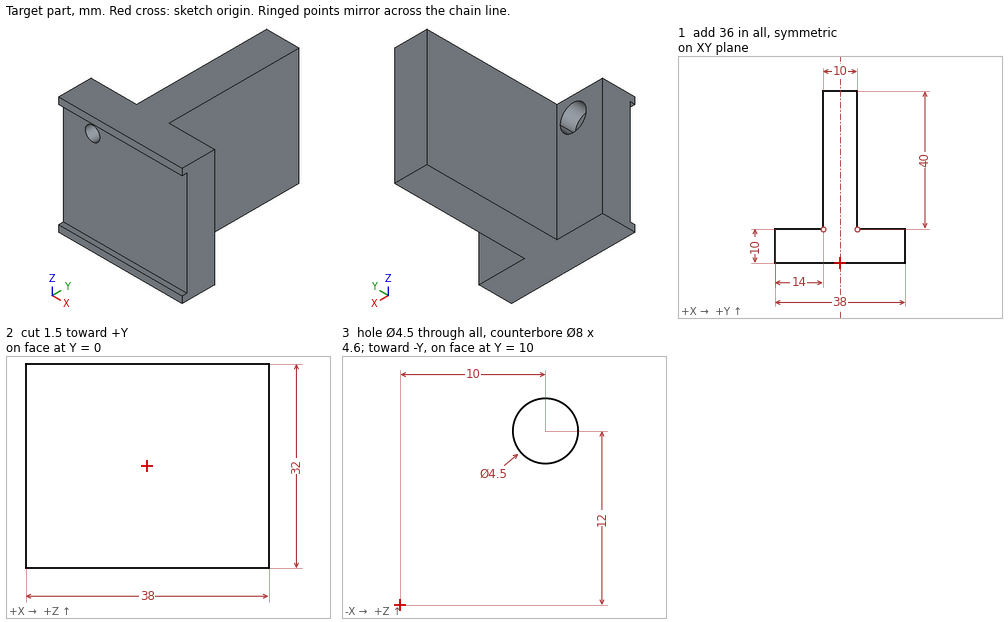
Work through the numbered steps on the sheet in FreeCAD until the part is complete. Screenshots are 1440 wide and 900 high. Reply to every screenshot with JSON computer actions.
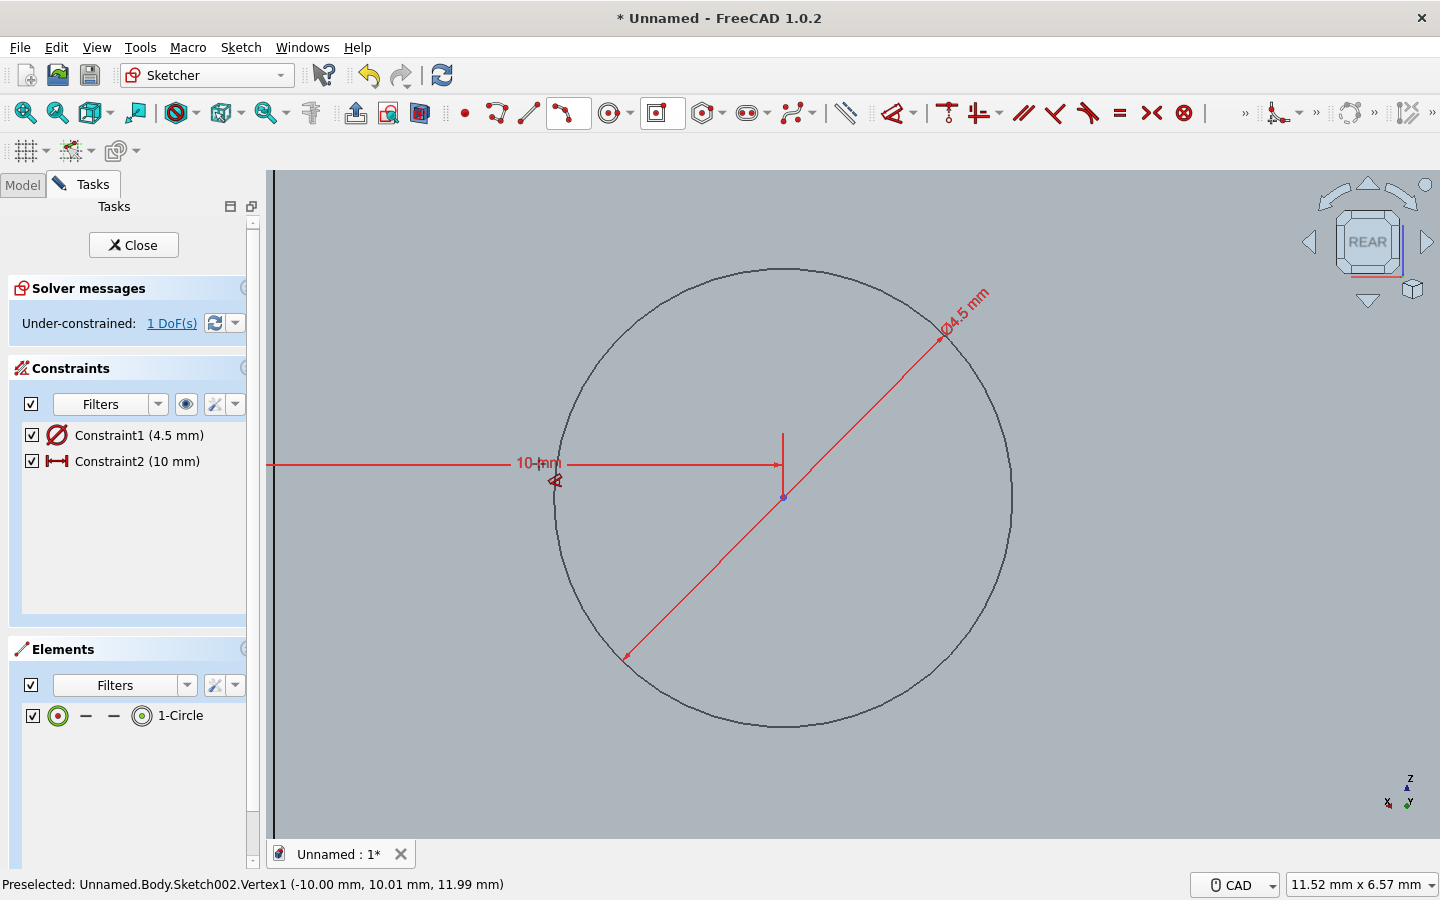
{"action": "left_click", "coordinate": [783, 498]}
{"action": "left_click", "coordinate": [817, 655]}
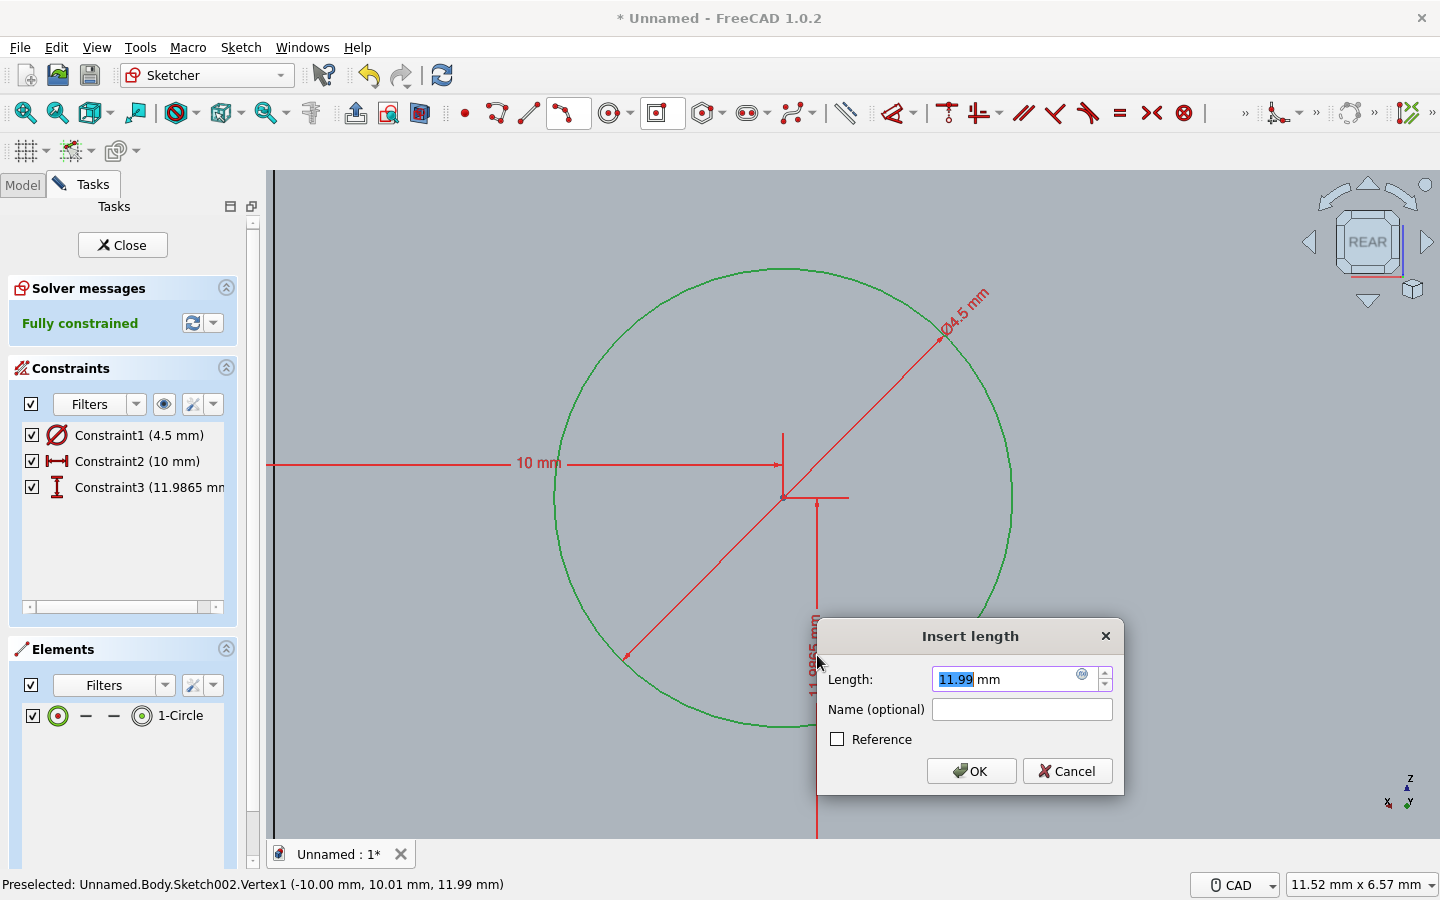
{"action": "type", "text": "12"}
{"action": "key", "text": "Return"}
{"action": "key", "text": "Escape"}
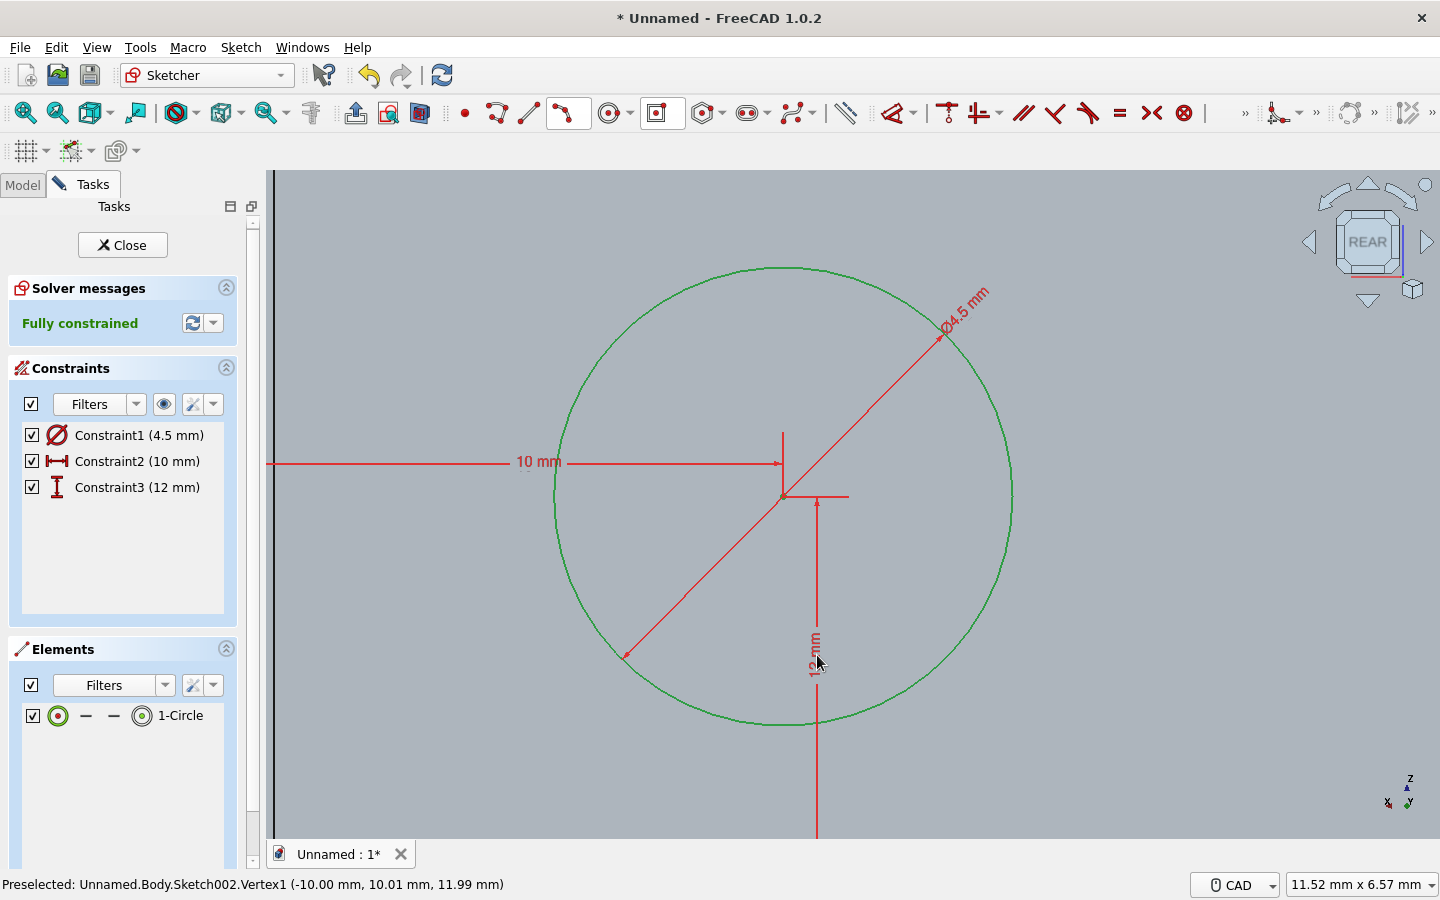
{"action": "left_click", "coordinate": [123, 245]}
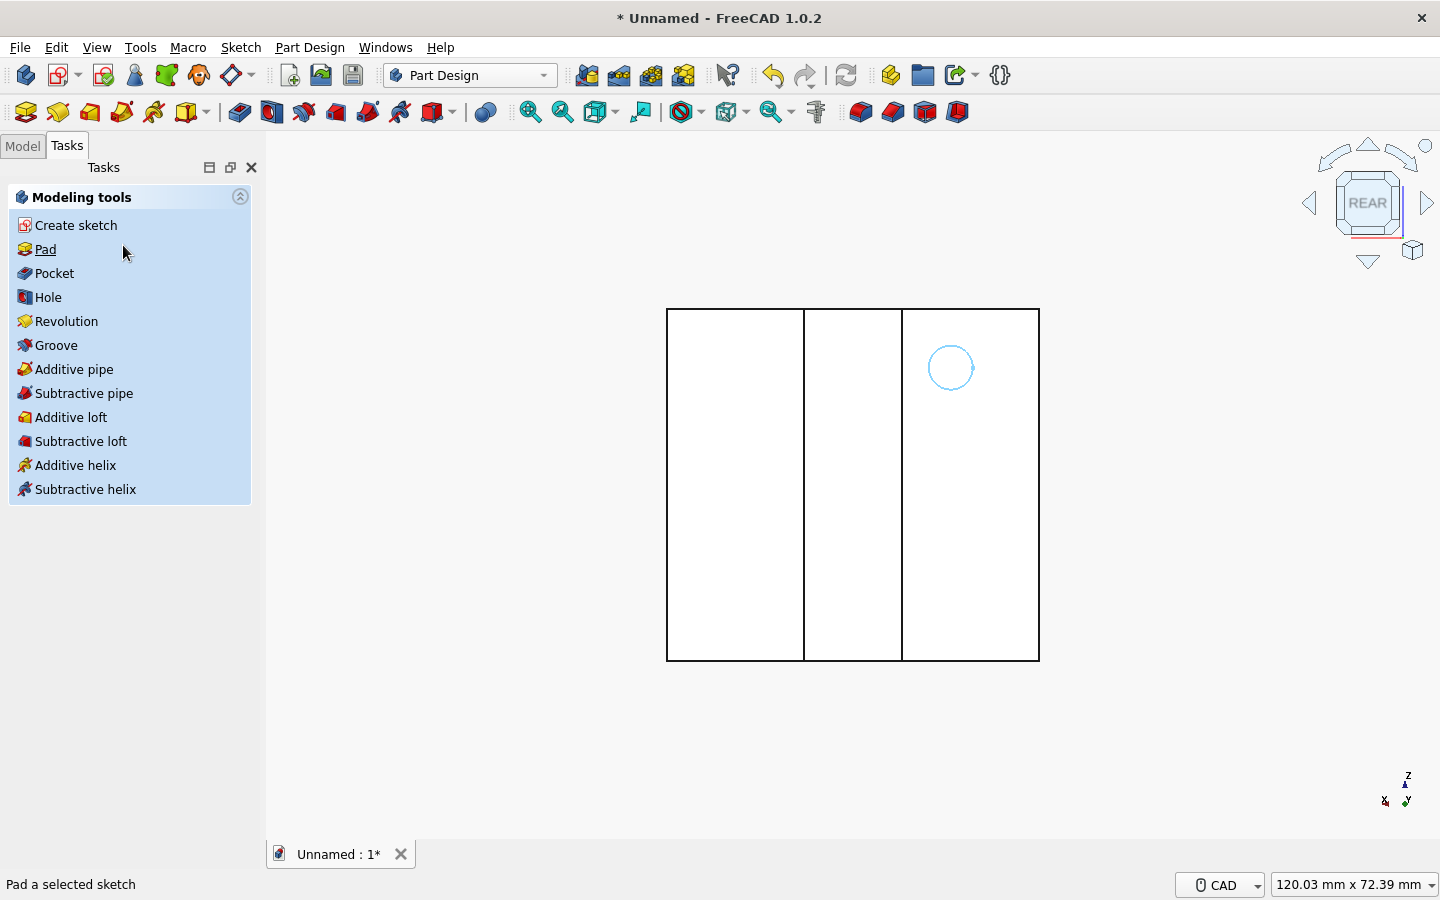
{"action": "left_click", "coordinate": [272, 112]}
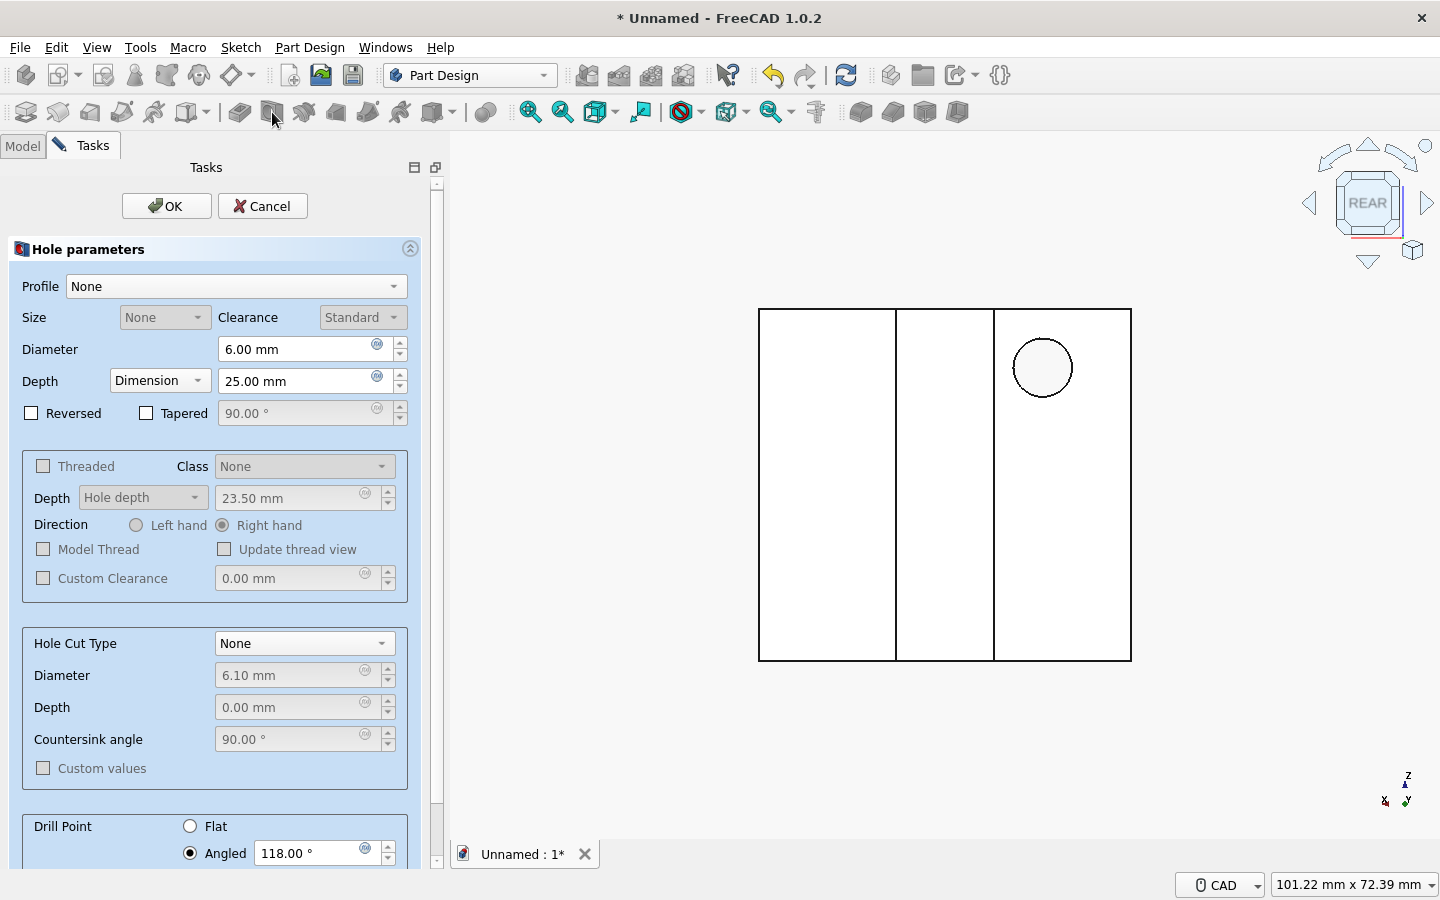
{"action": "triple_click", "coordinate": [305, 349]}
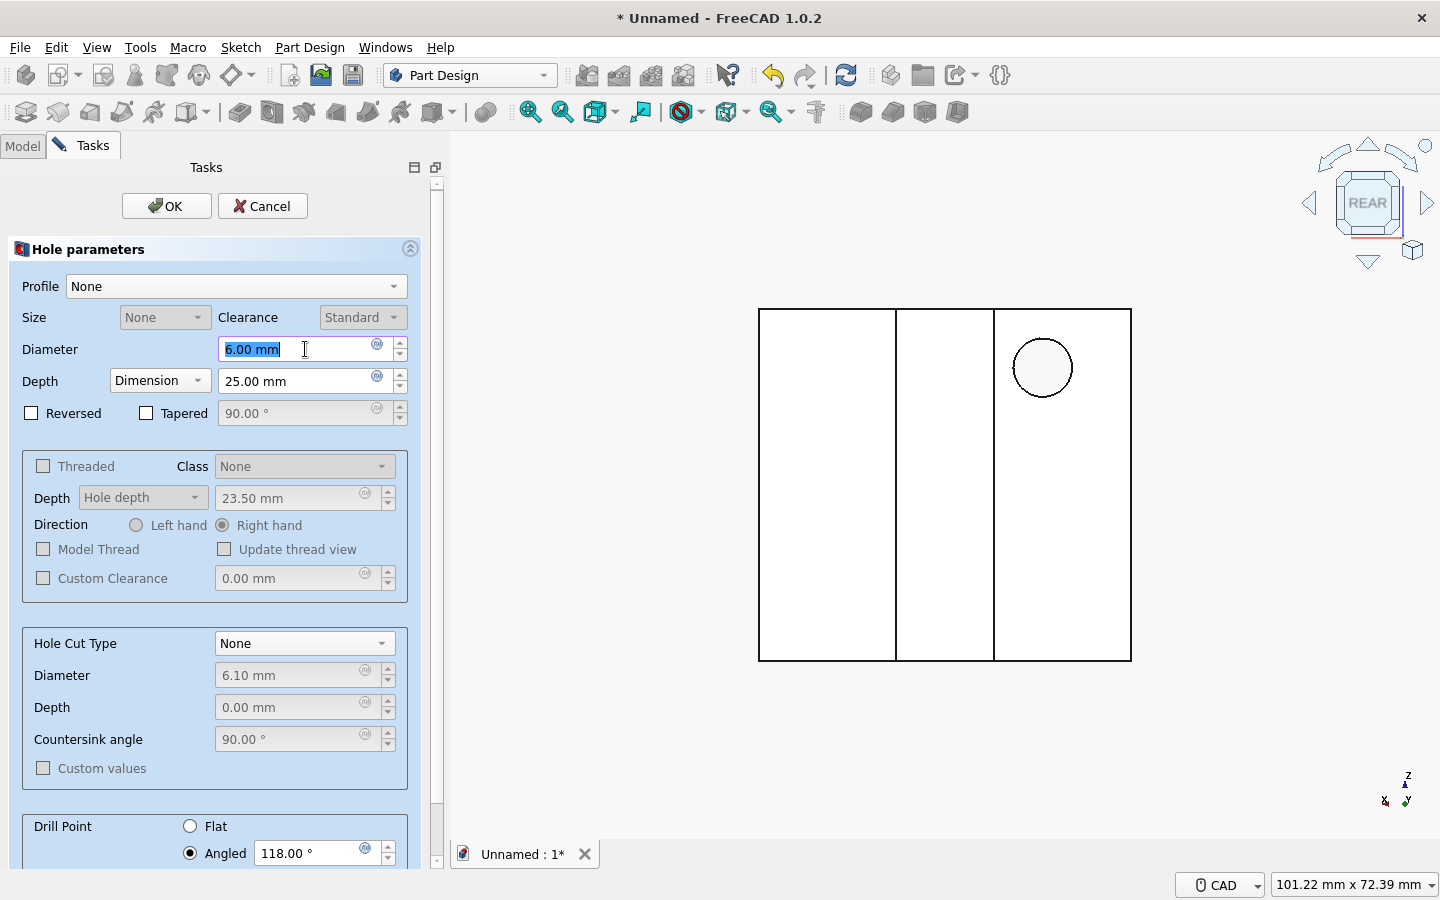
{"action": "type", "text": "4.5"}
{"action": "key", "text": "Tab"}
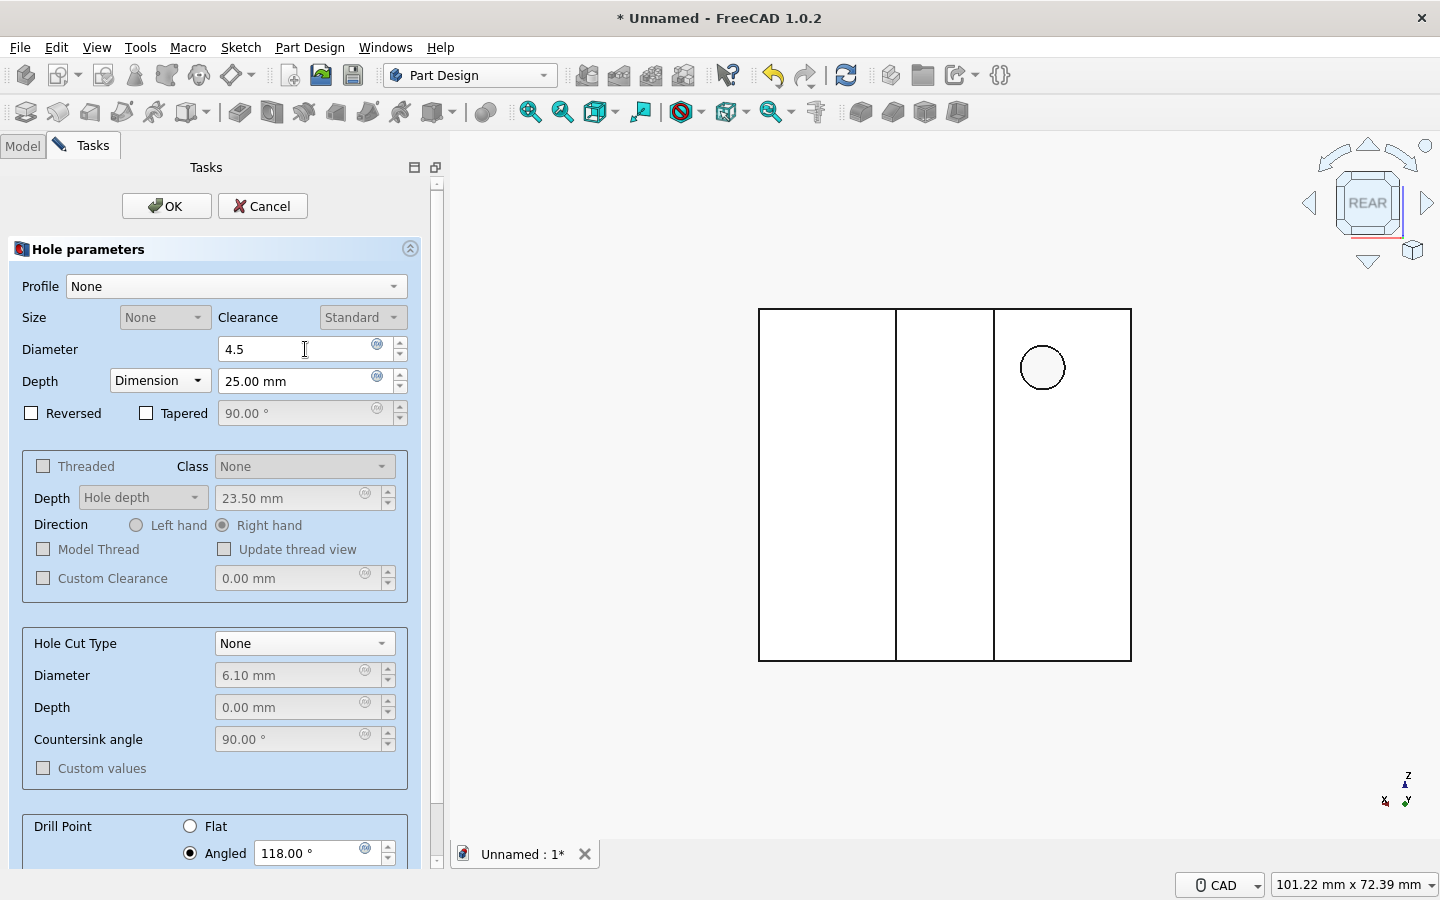
{"action": "left_click", "coordinate": [161, 380]}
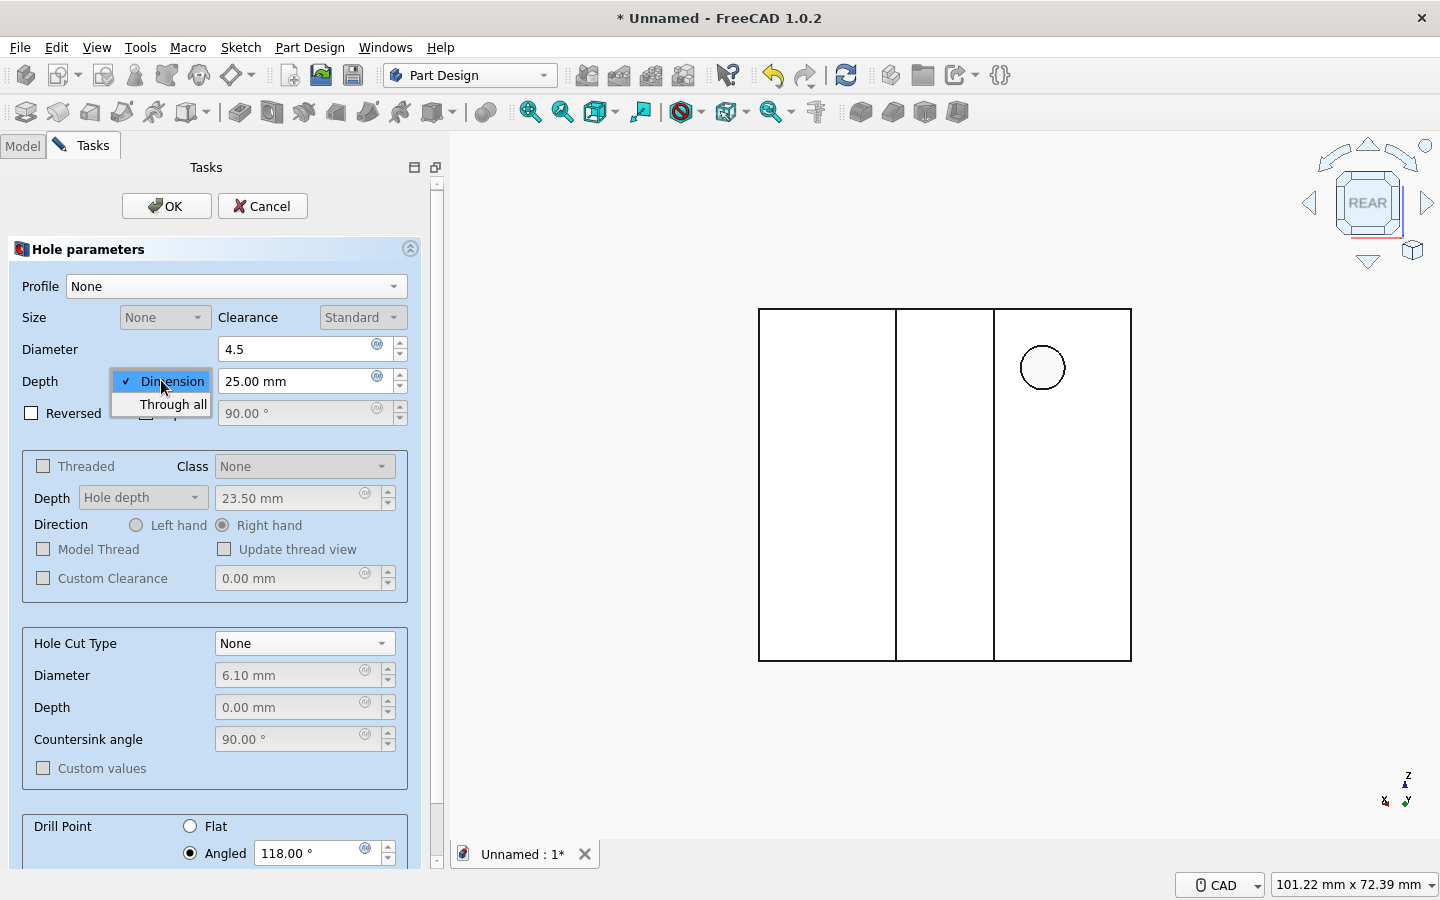
{"action": "left_click", "coordinate": [160, 404]}